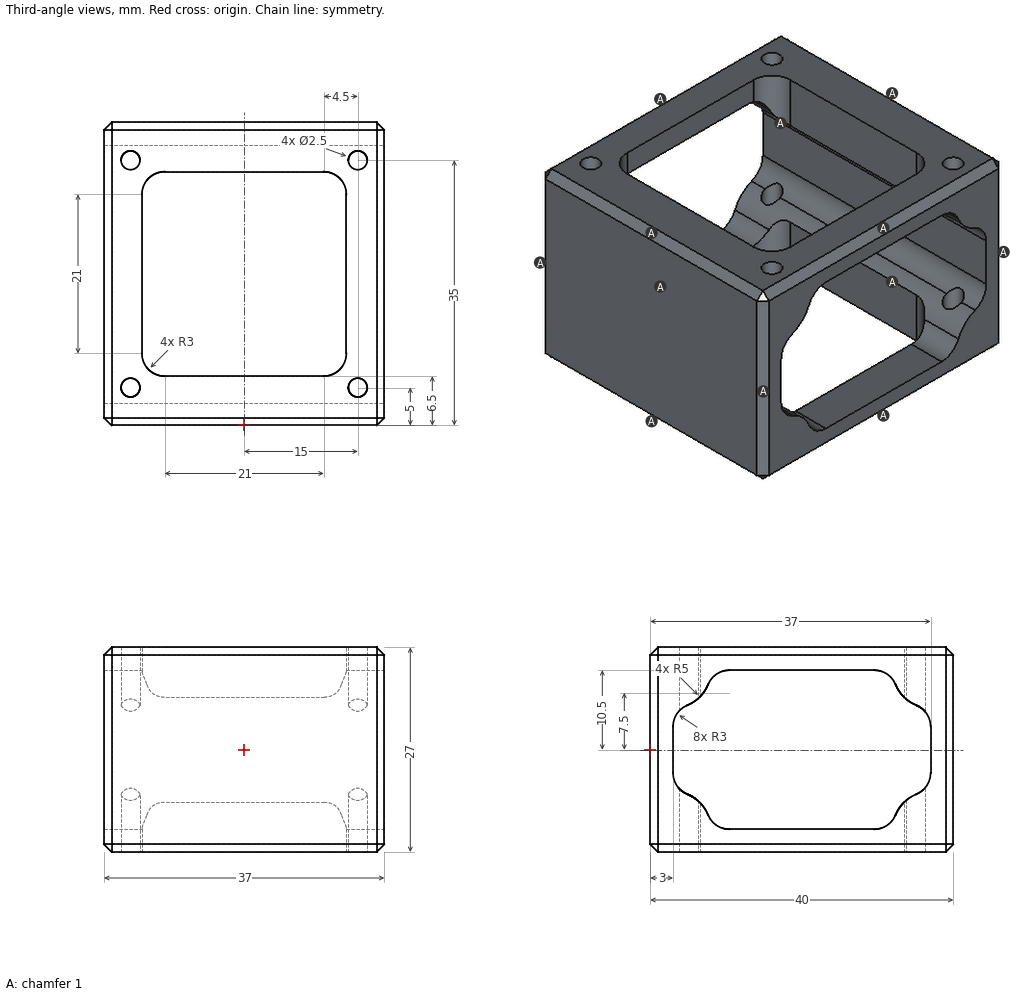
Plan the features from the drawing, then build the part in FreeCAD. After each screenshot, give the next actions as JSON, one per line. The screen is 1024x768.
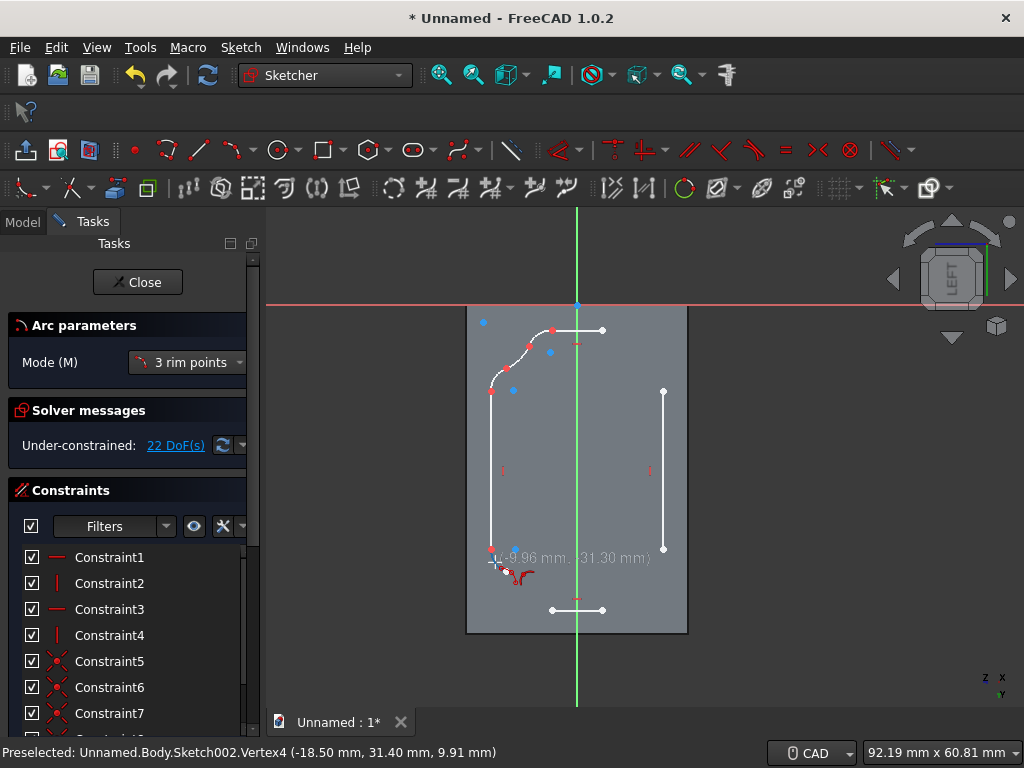
{"action": "left_click", "coordinate": [506, 572]}
{"action": "left_click", "coordinate": [529, 594]}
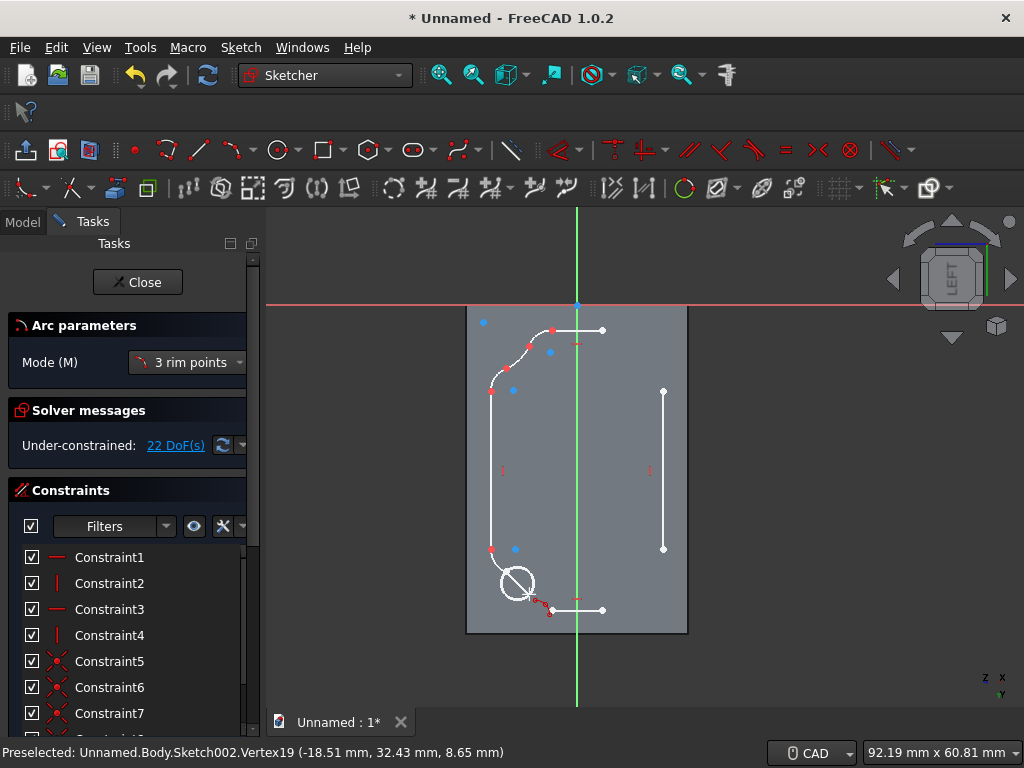
{"action": "scroll", "coordinate": [520, 581], "scroll_direction": "up", "scroll_amount": 8}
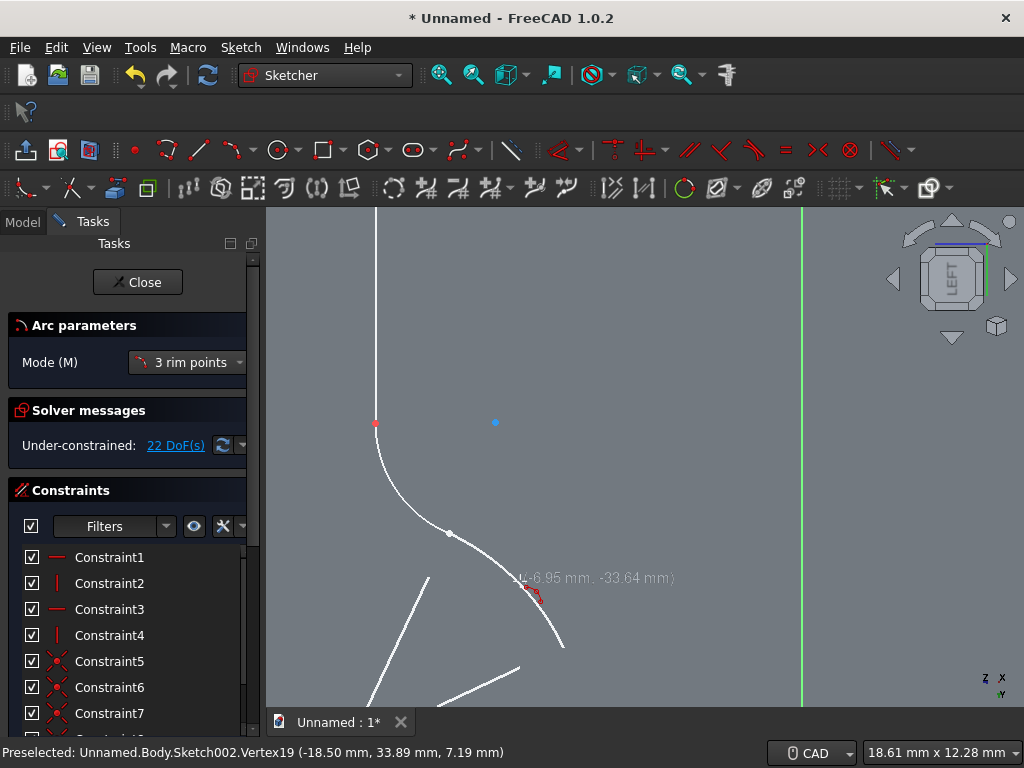
{"action": "left_click", "coordinate": [518, 576]}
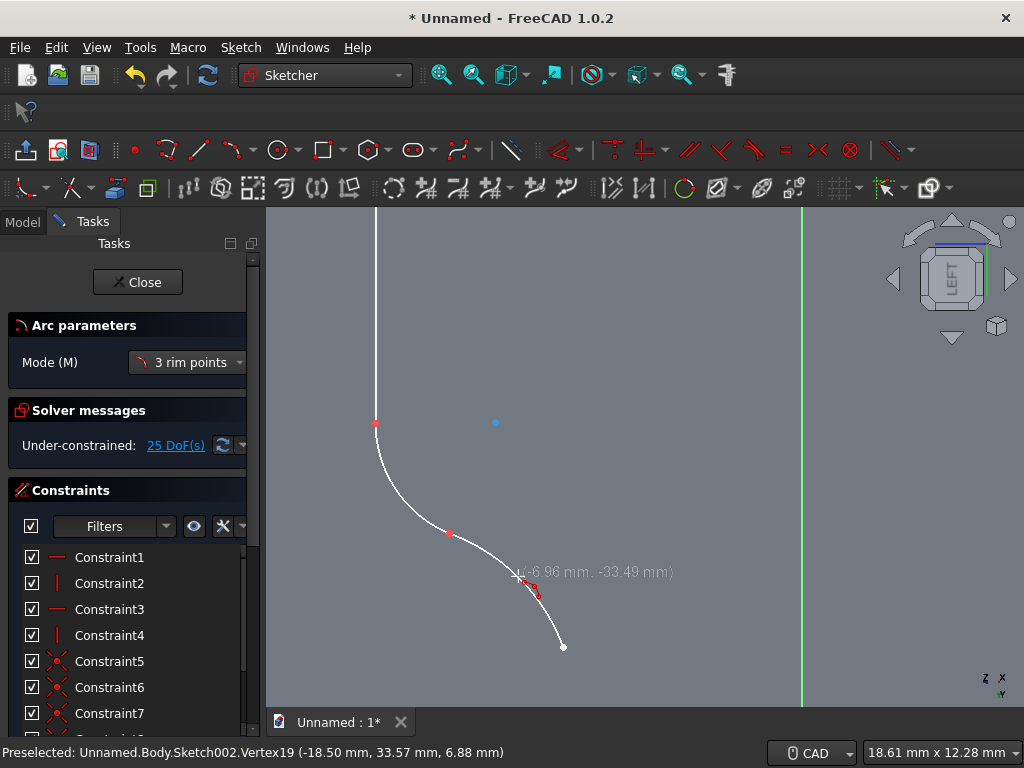
{"action": "scroll", "coordinate": [520, 581], "scroll_direction": "down", "scroll_amount": 8}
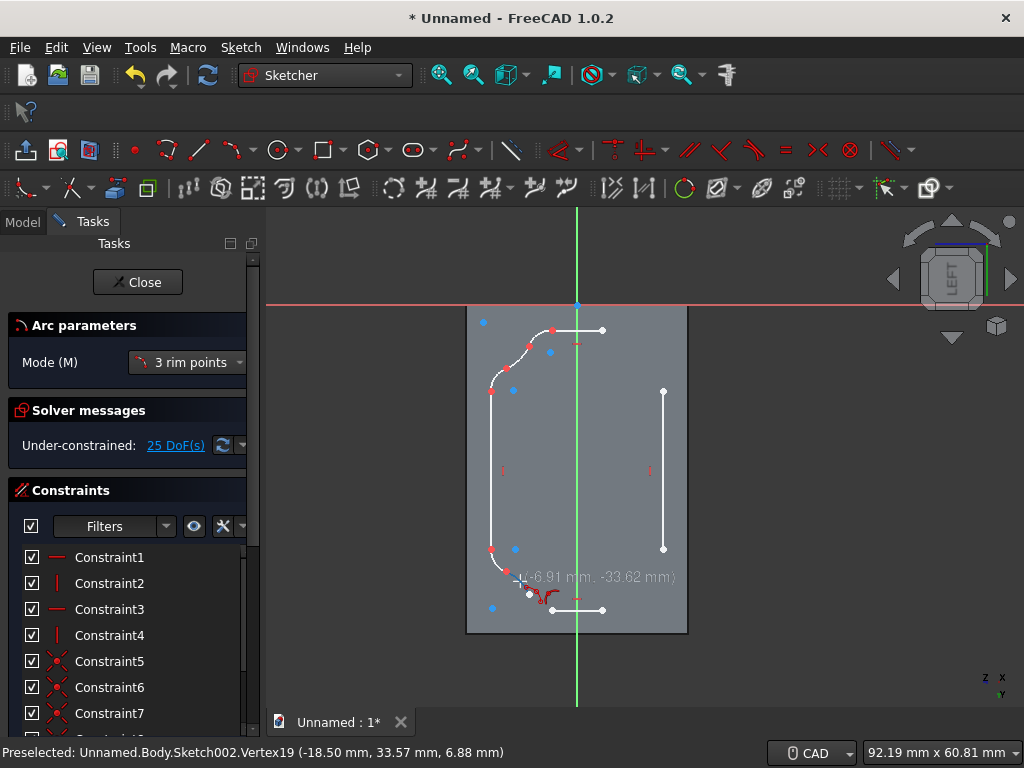
{"action": "left_click", "coordinate": [529, 595]}
{"action": "left_click", "coordinate": [552, 611]}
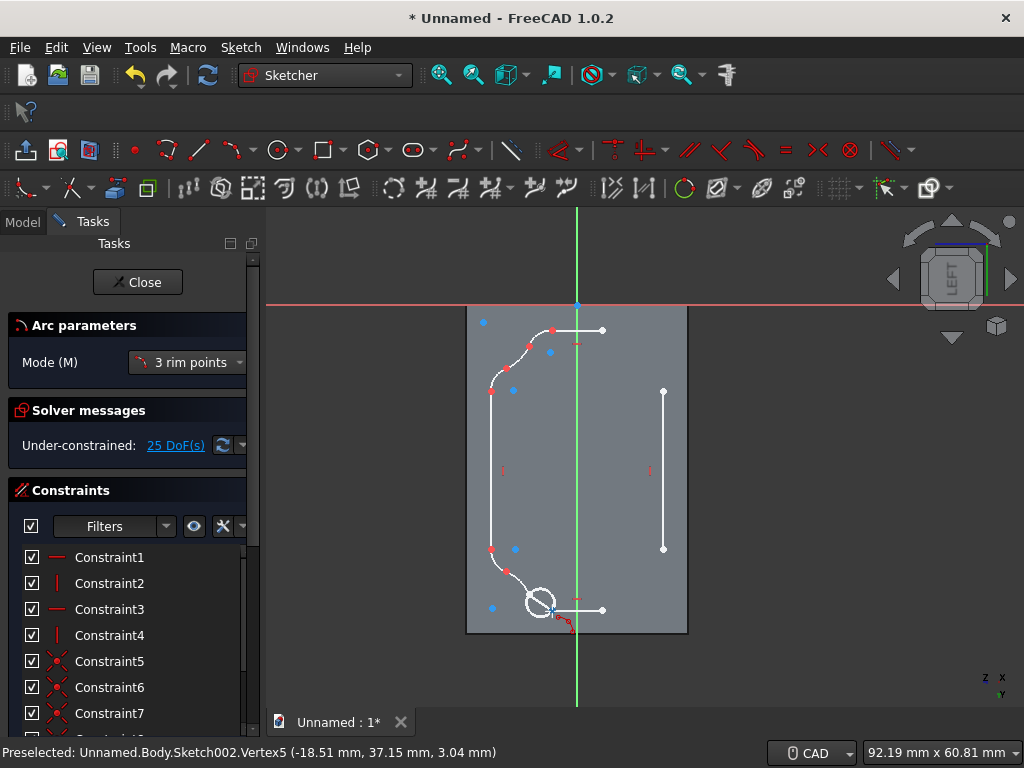
{"action": "scroll", "coordinate": [538, 605], "scroll_direction": "up", "scroll_amount": 7}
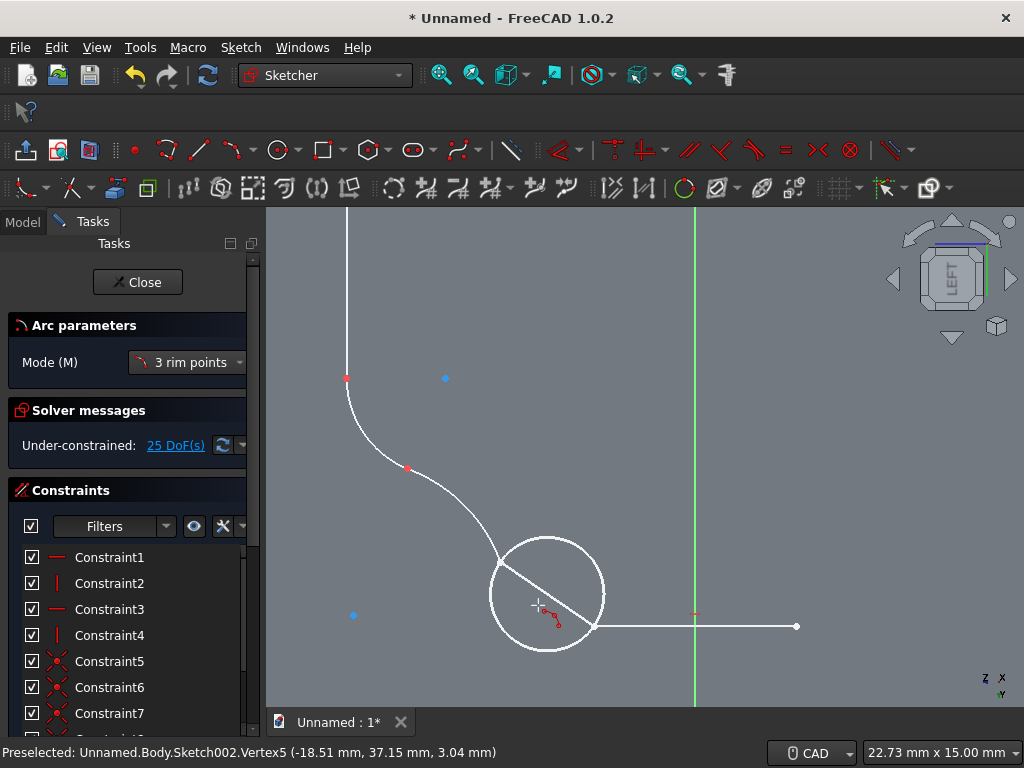
{"action": "left_click", "coordinate": [537, 604]}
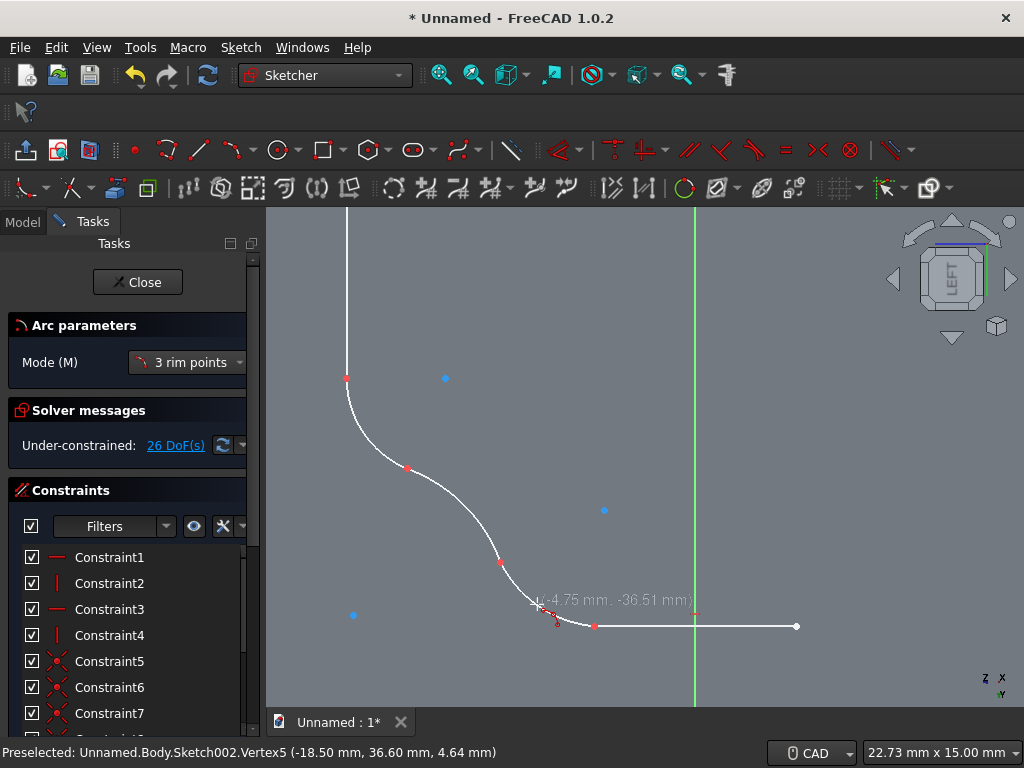
{"action": "scroll", "coordinate": [538, 605], "scroll_direction": "down", "scroll_amount": 7}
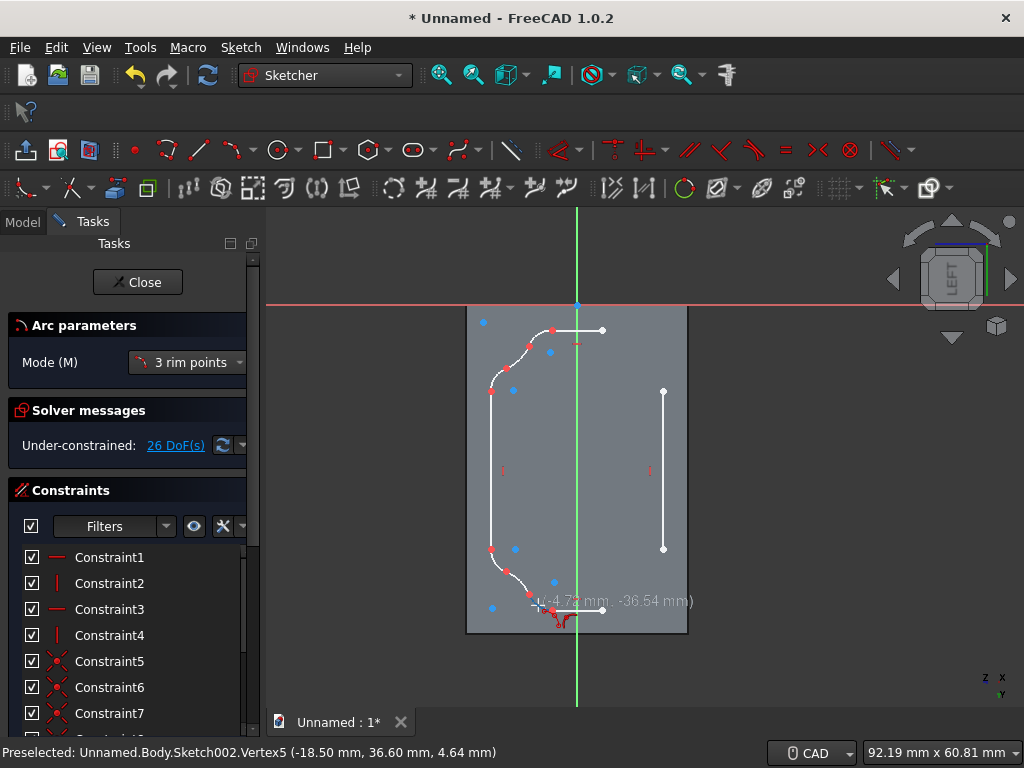
{"action": "left_click", "coordinate": [602, 611]}
{"action": "left_click", "coordinate": [625, 594]}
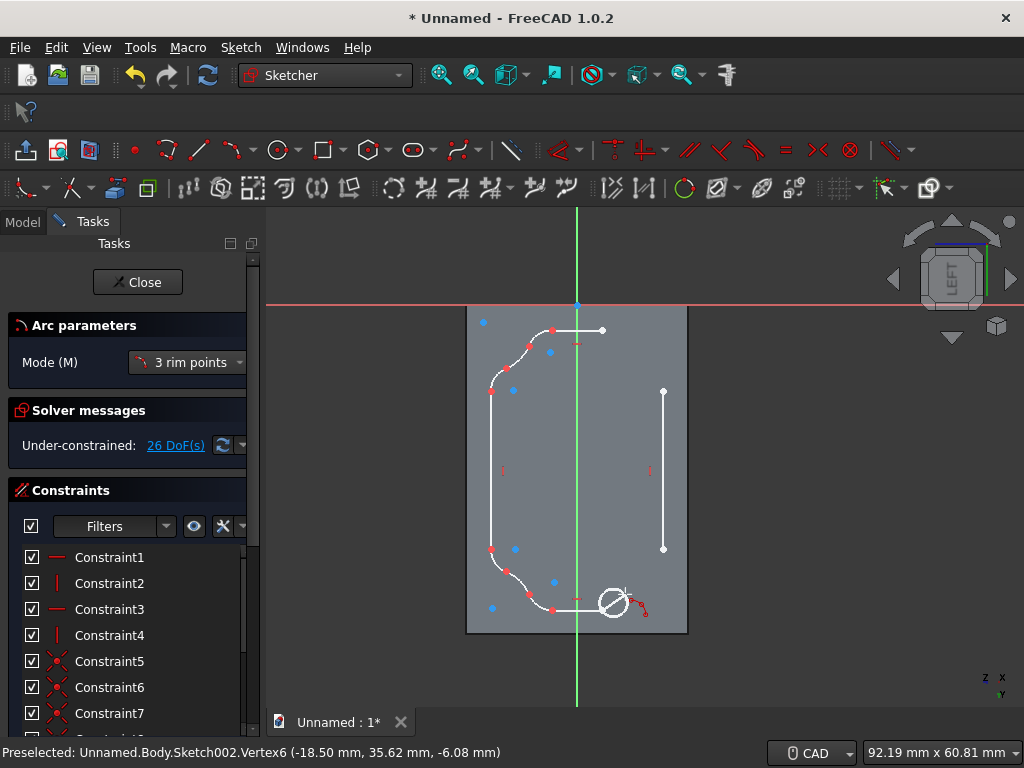
{"action": "scroll", "coordinate": [616, 605], "scroll_direction": "up", "scroll_amount": 7}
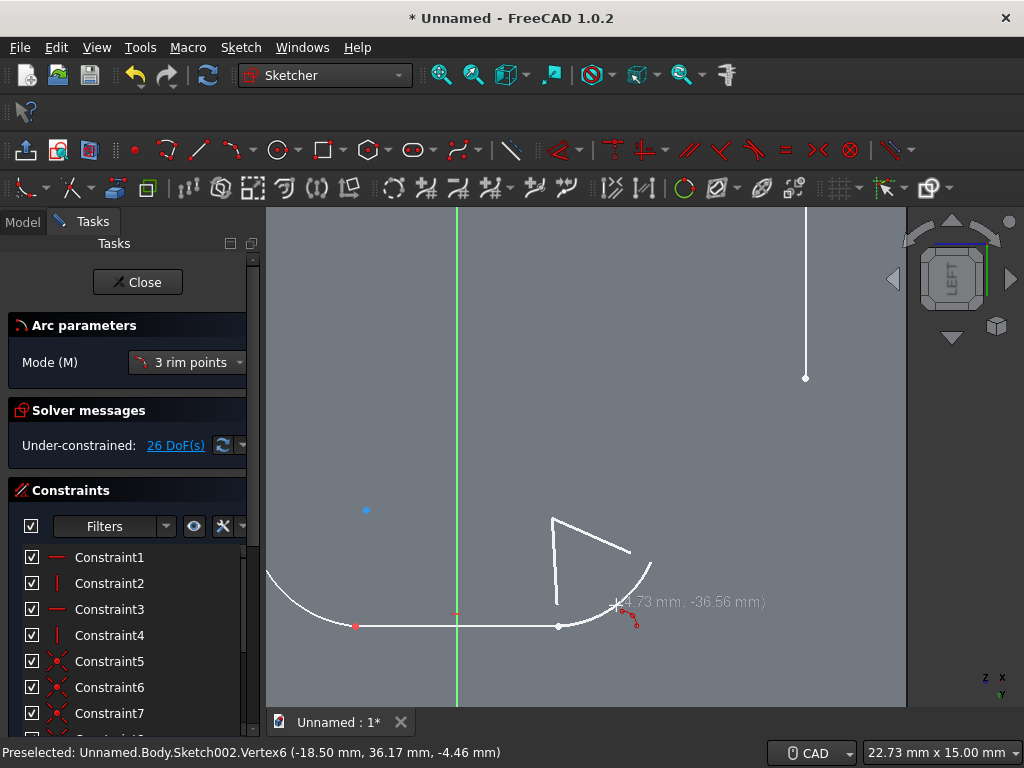
{"action": "left_click", "coordinate": [616, 604]}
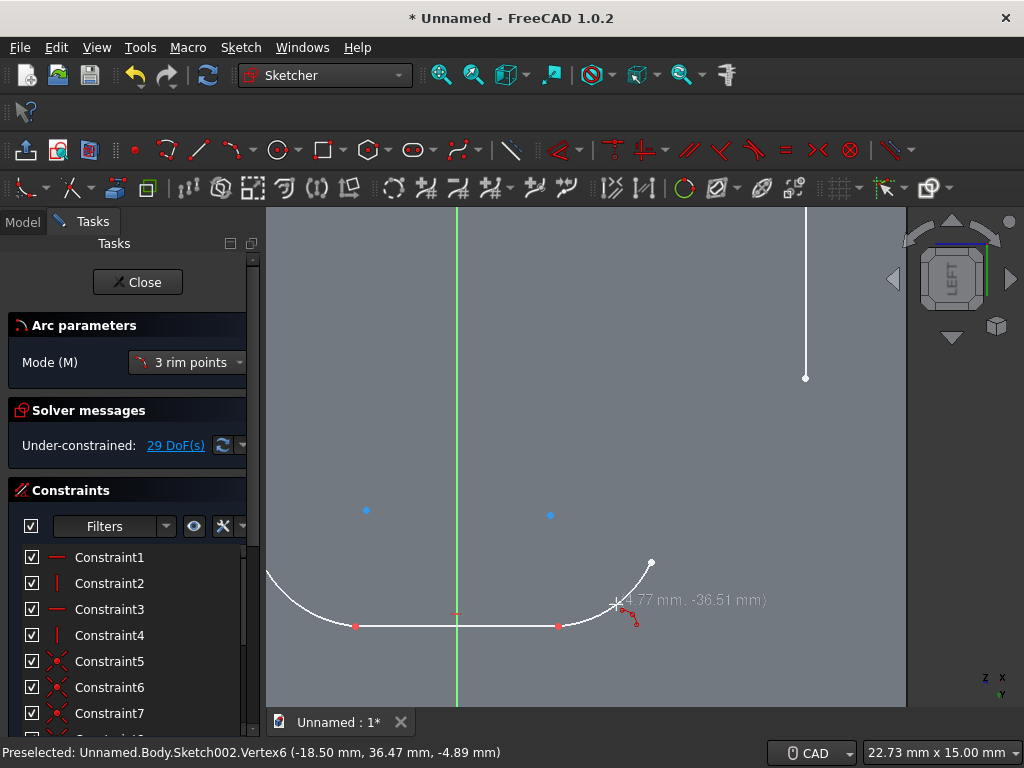
{"action": "scroll", "coordinate": [616, 605], "scroll_direction": "down", "scroll_amount": 7}